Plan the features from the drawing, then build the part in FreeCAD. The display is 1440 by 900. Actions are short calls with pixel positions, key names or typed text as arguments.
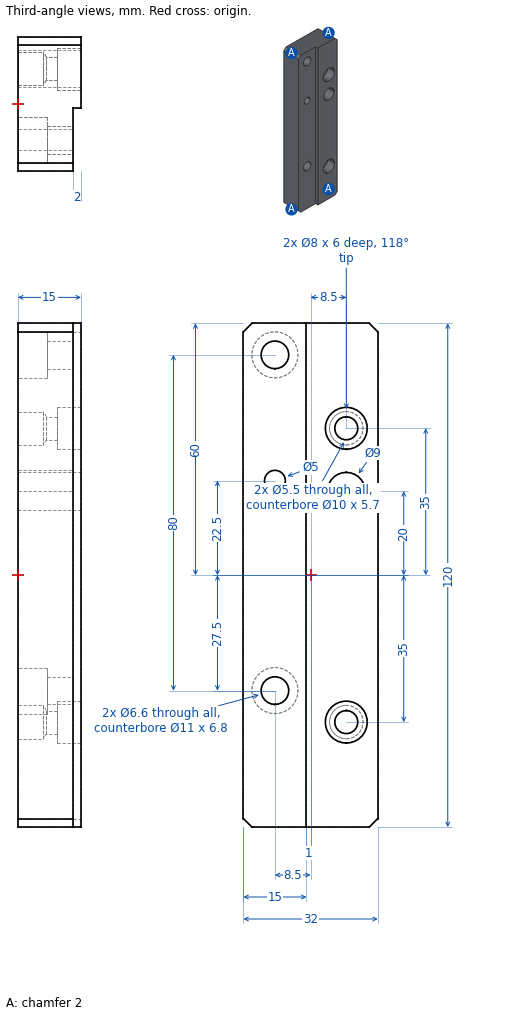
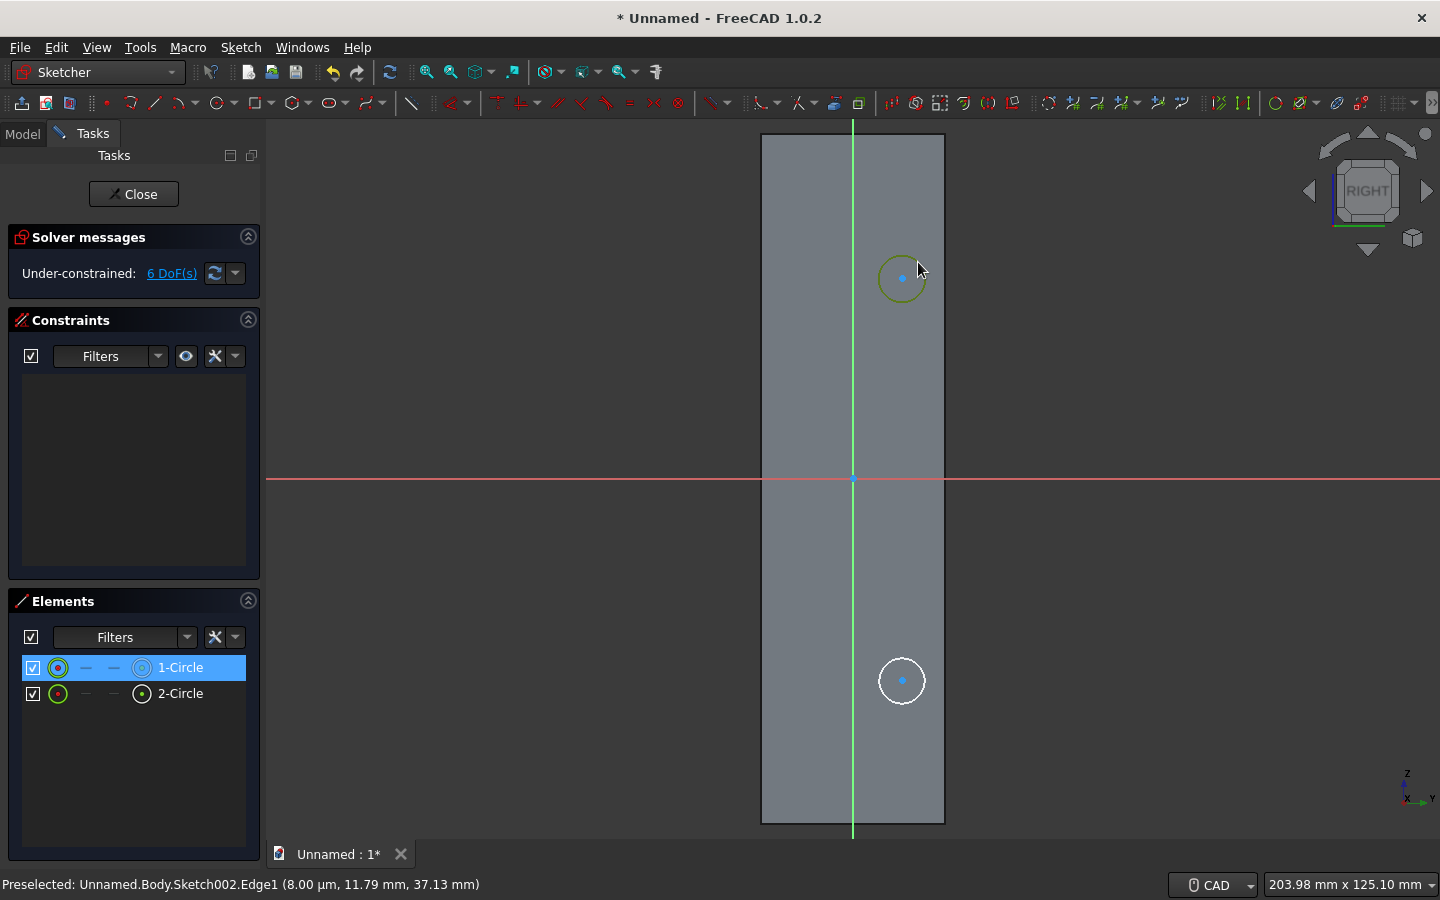
click(918, 665)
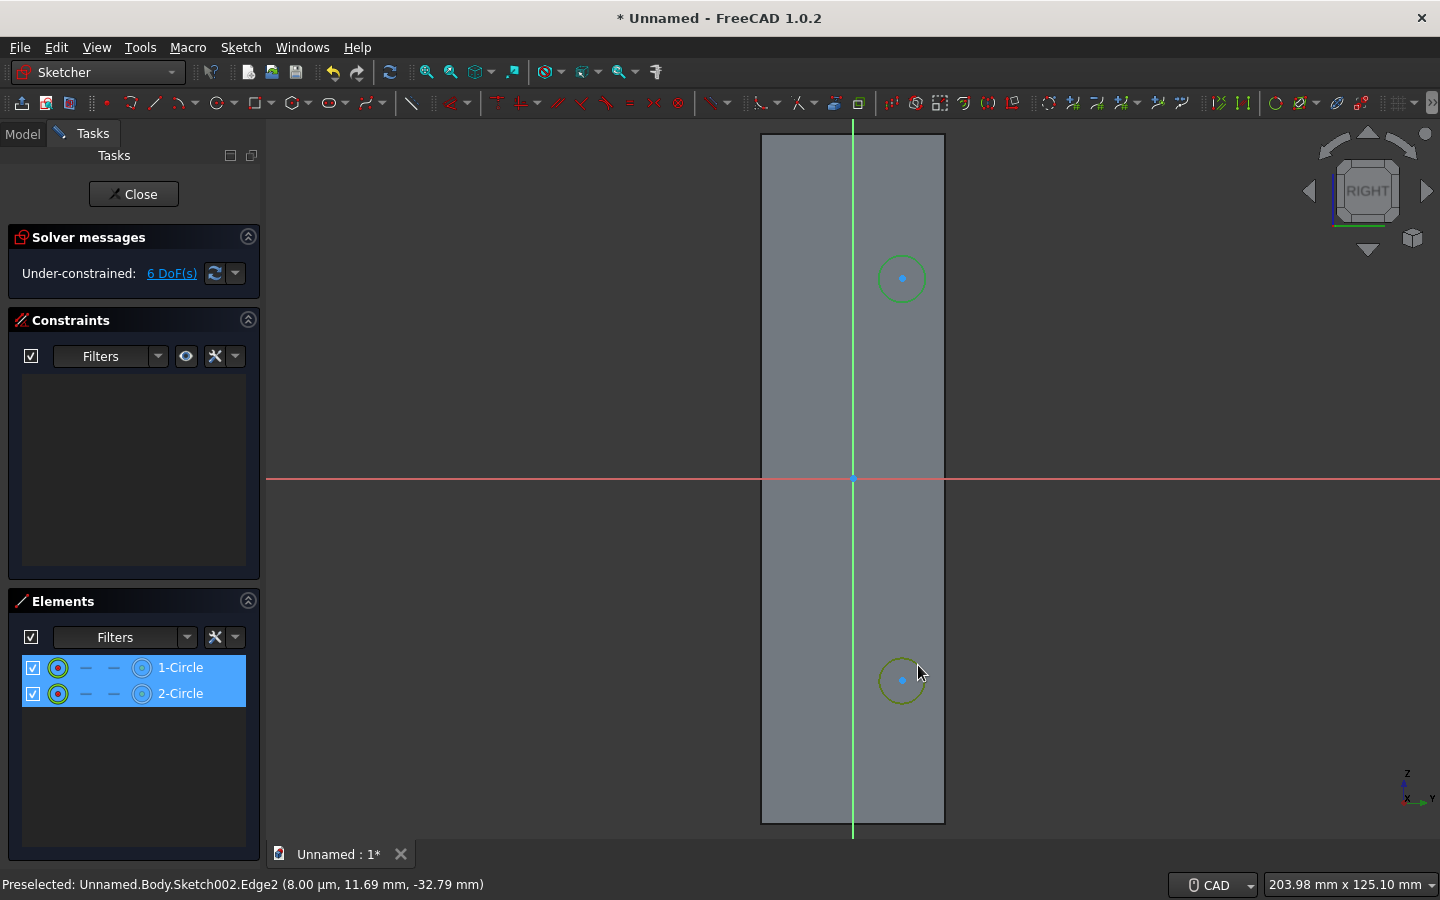
click(630, 104)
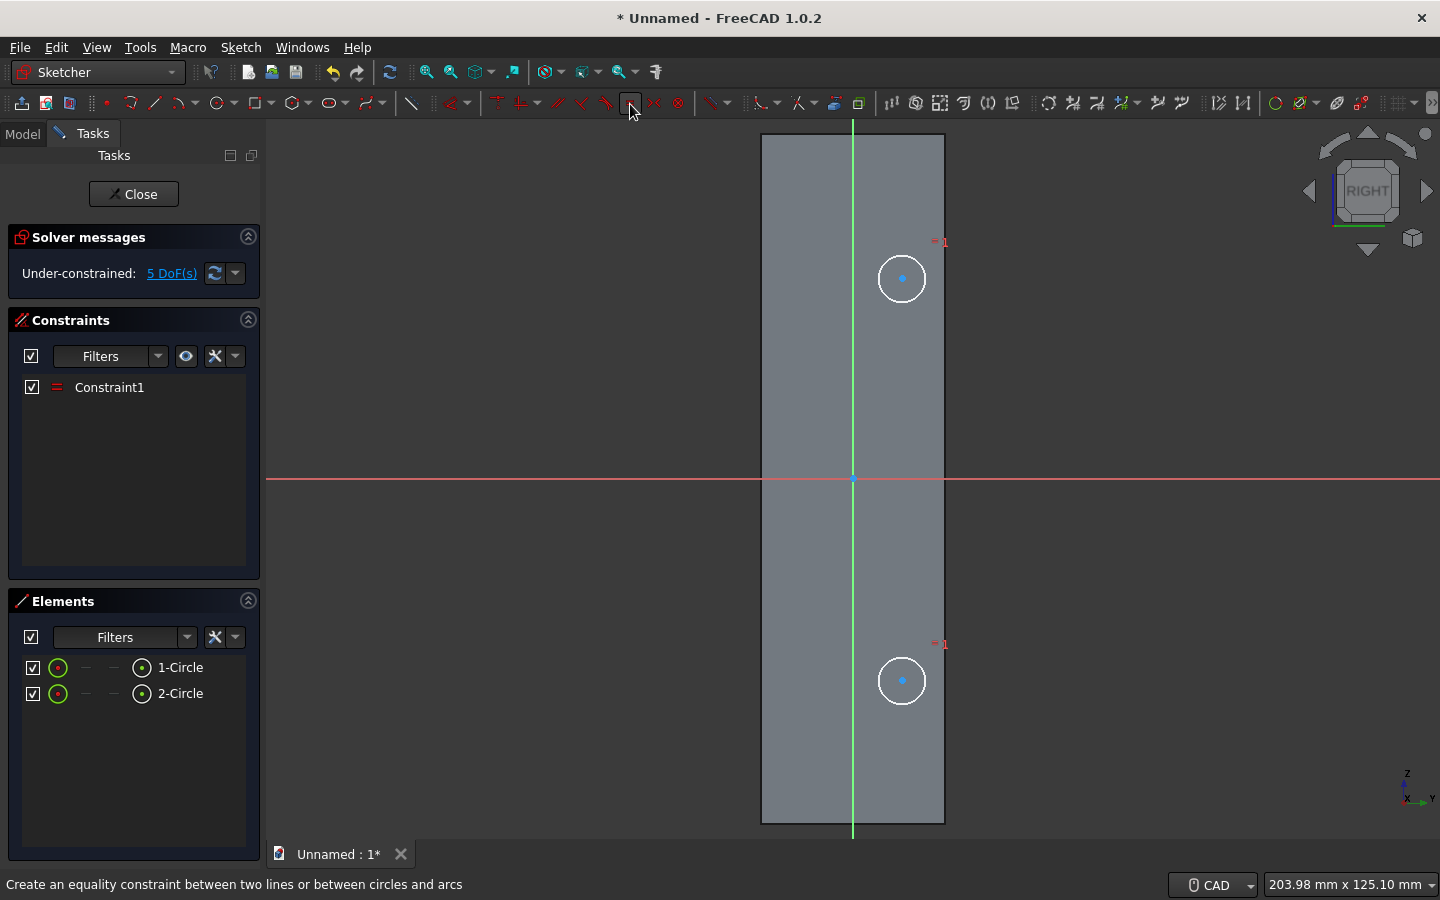
click(902, 279)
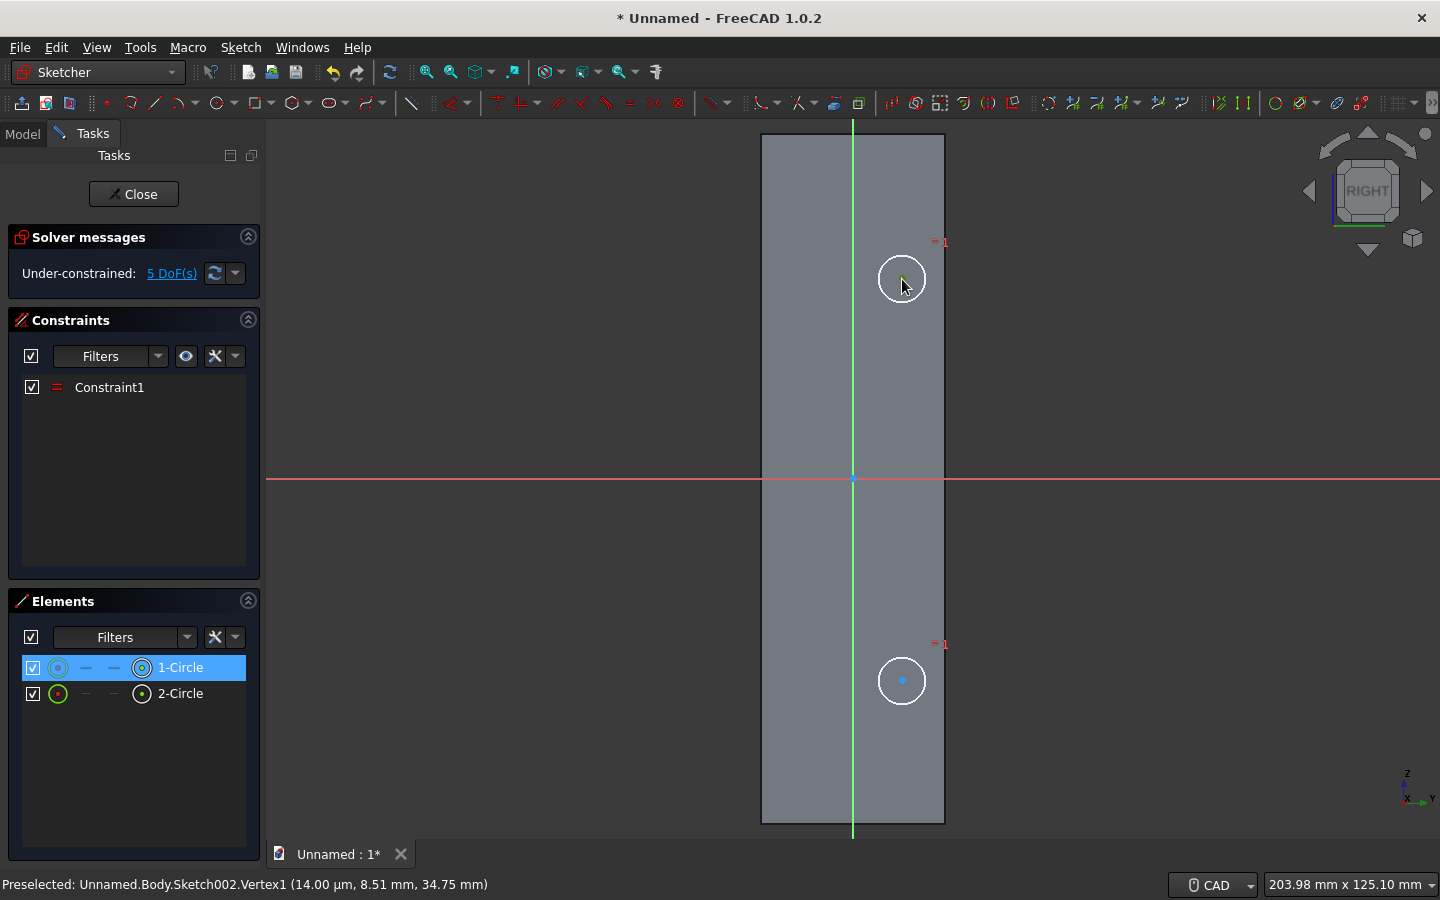
click(902, 681)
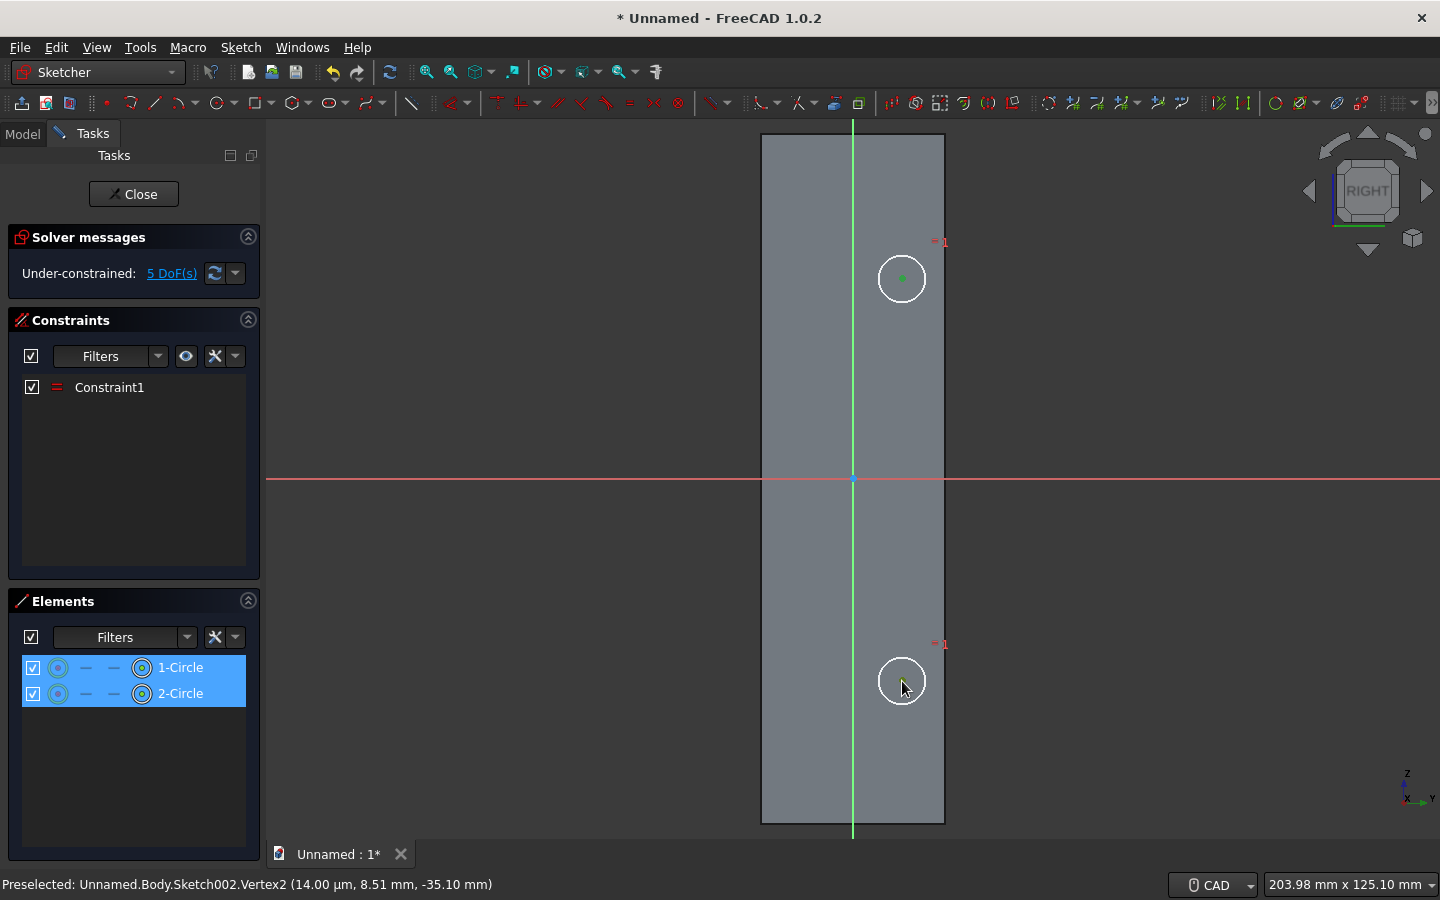
key(v)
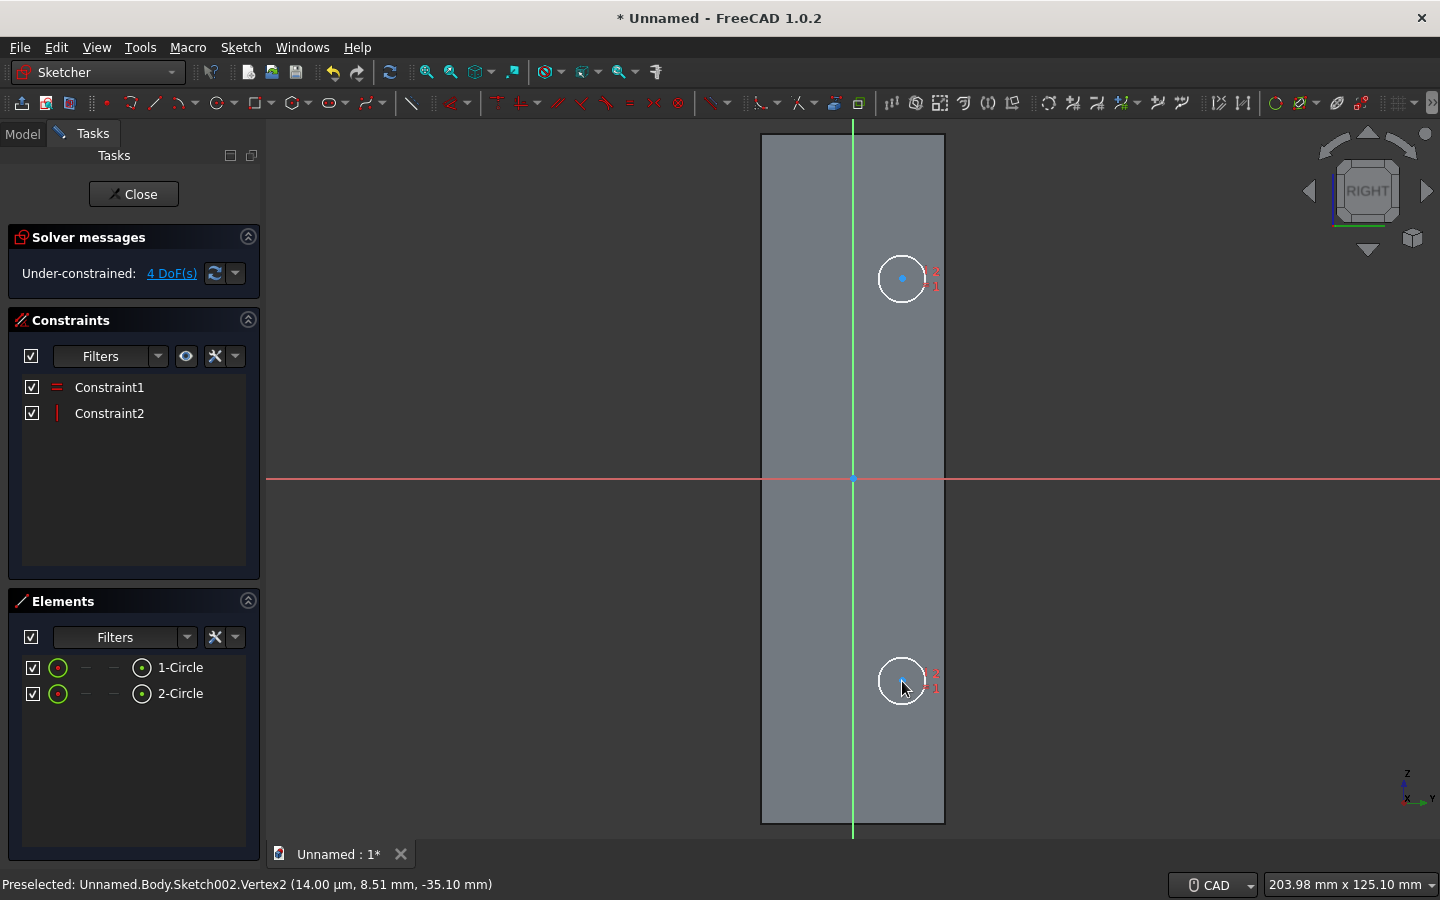
click(450, 104)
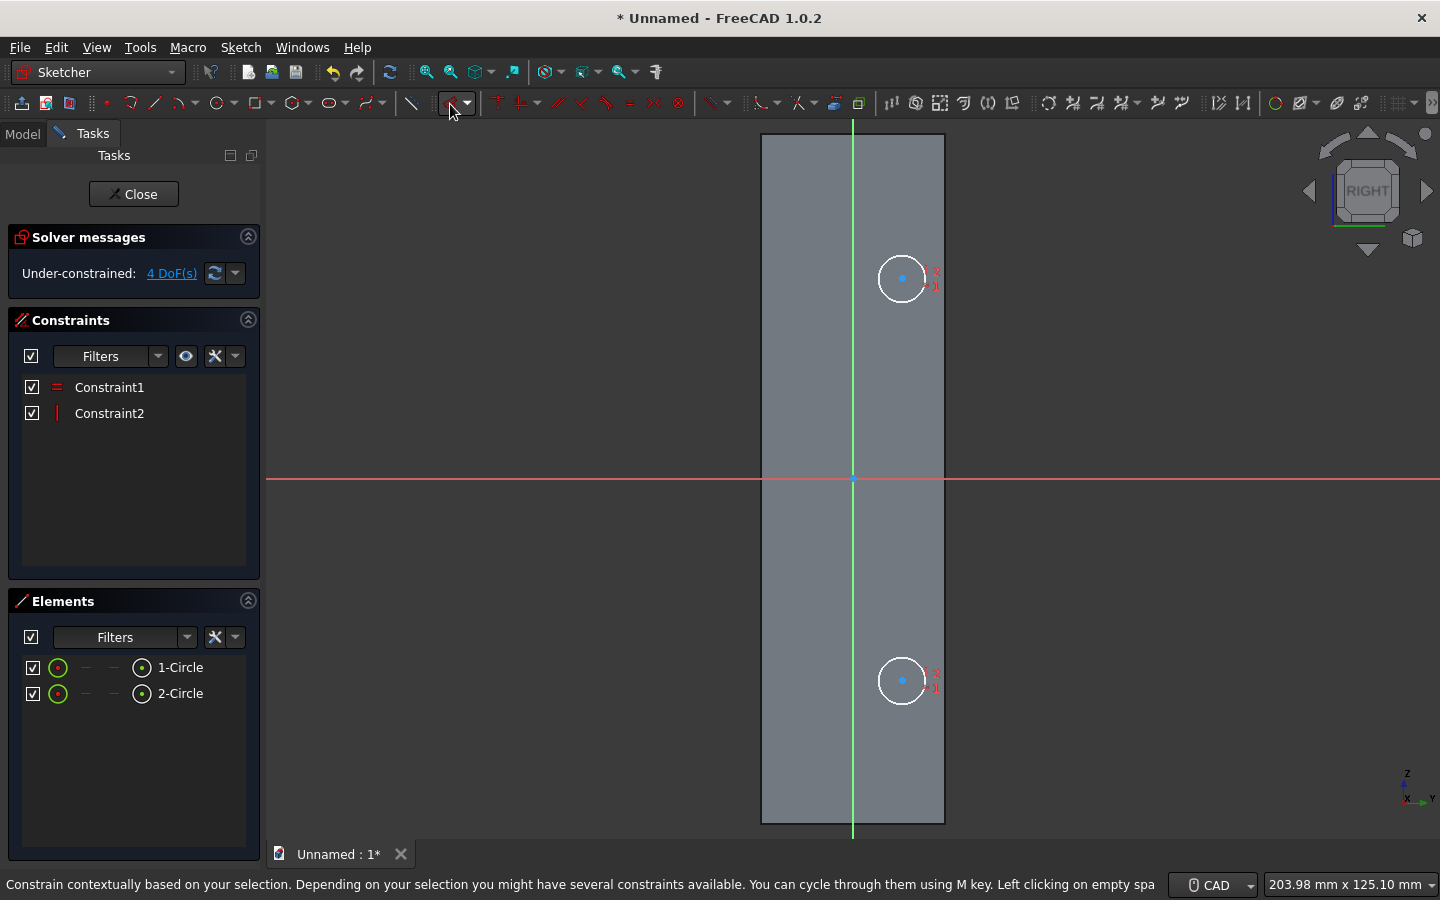
click(918, 262)
click(940, 239)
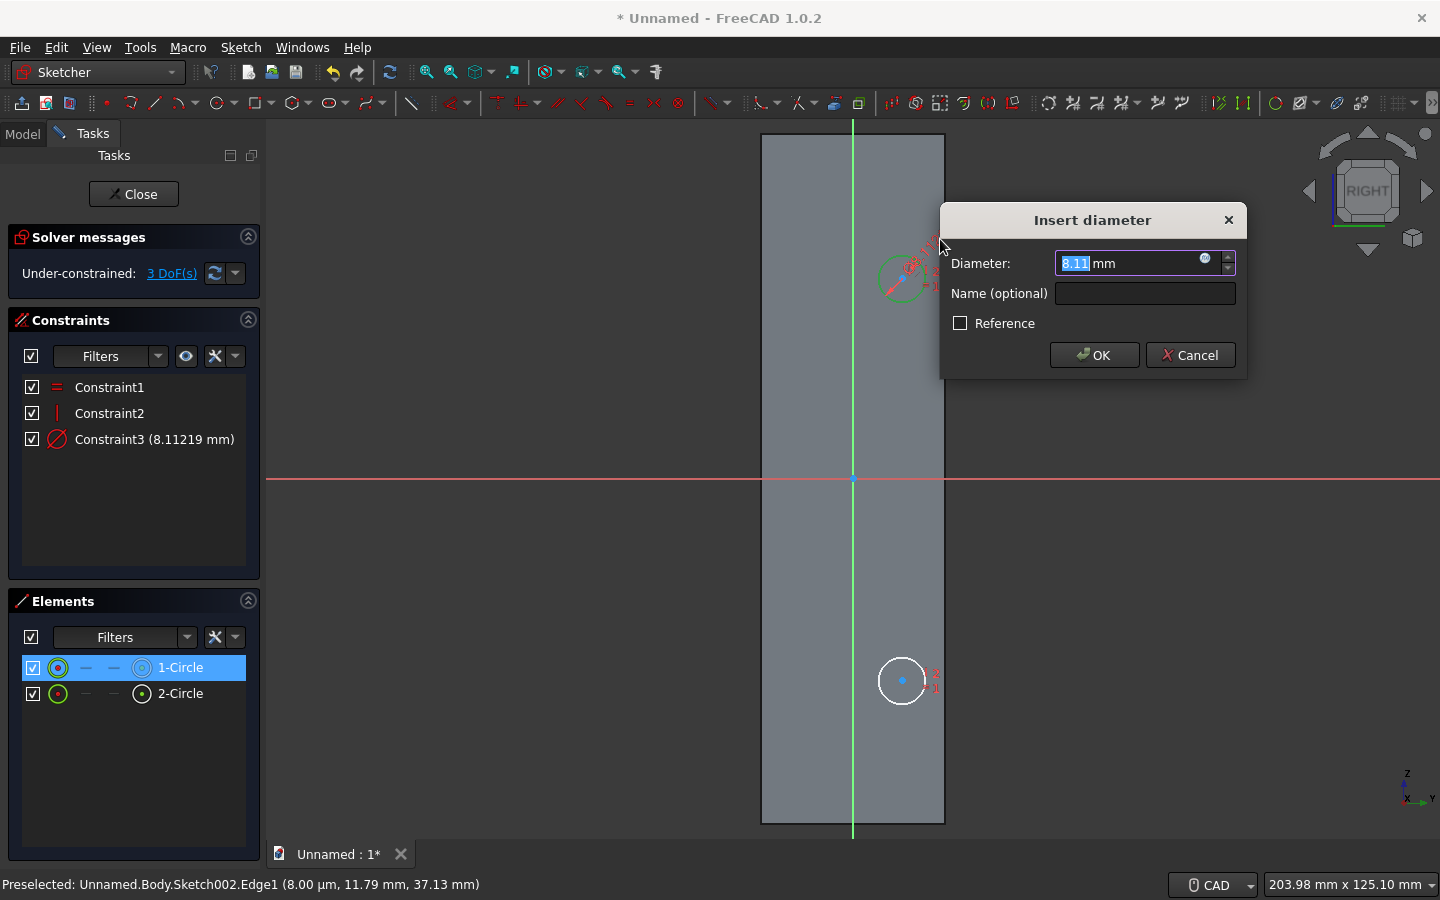
text(8)
key(Return)